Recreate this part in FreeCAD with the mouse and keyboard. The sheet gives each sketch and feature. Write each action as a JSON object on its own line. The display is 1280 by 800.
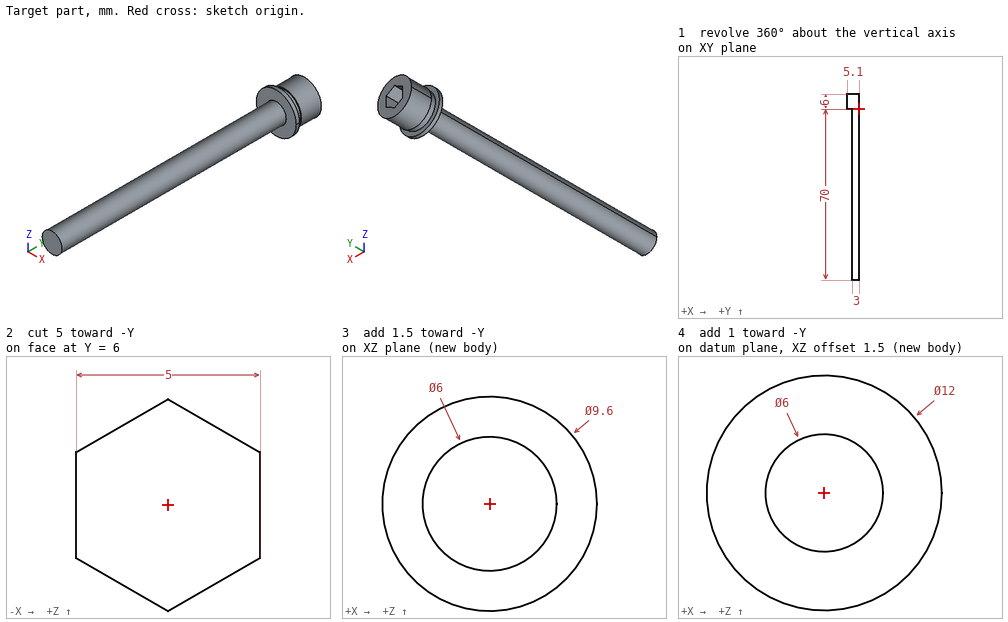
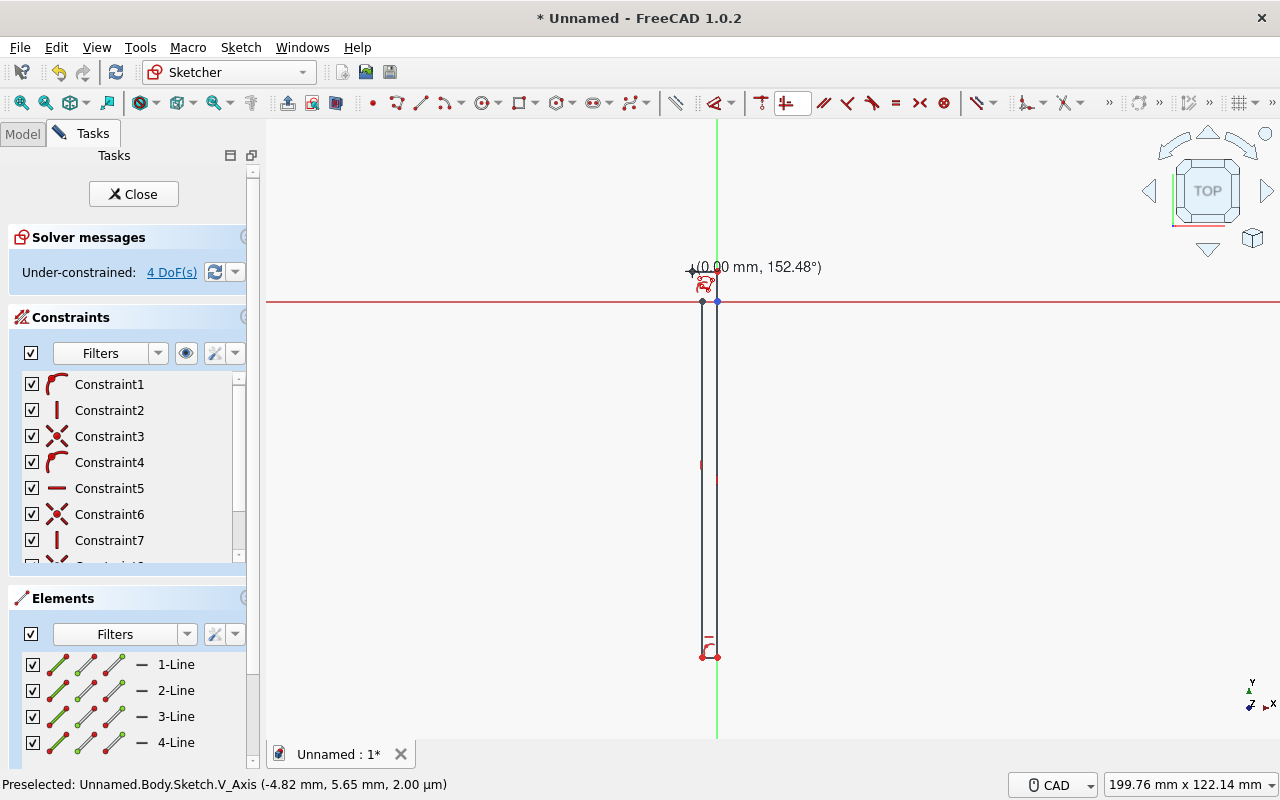
{"action": "scroll", "coordinate": [692, 302], "scroll_direction": "up", "scroll_amount": 2}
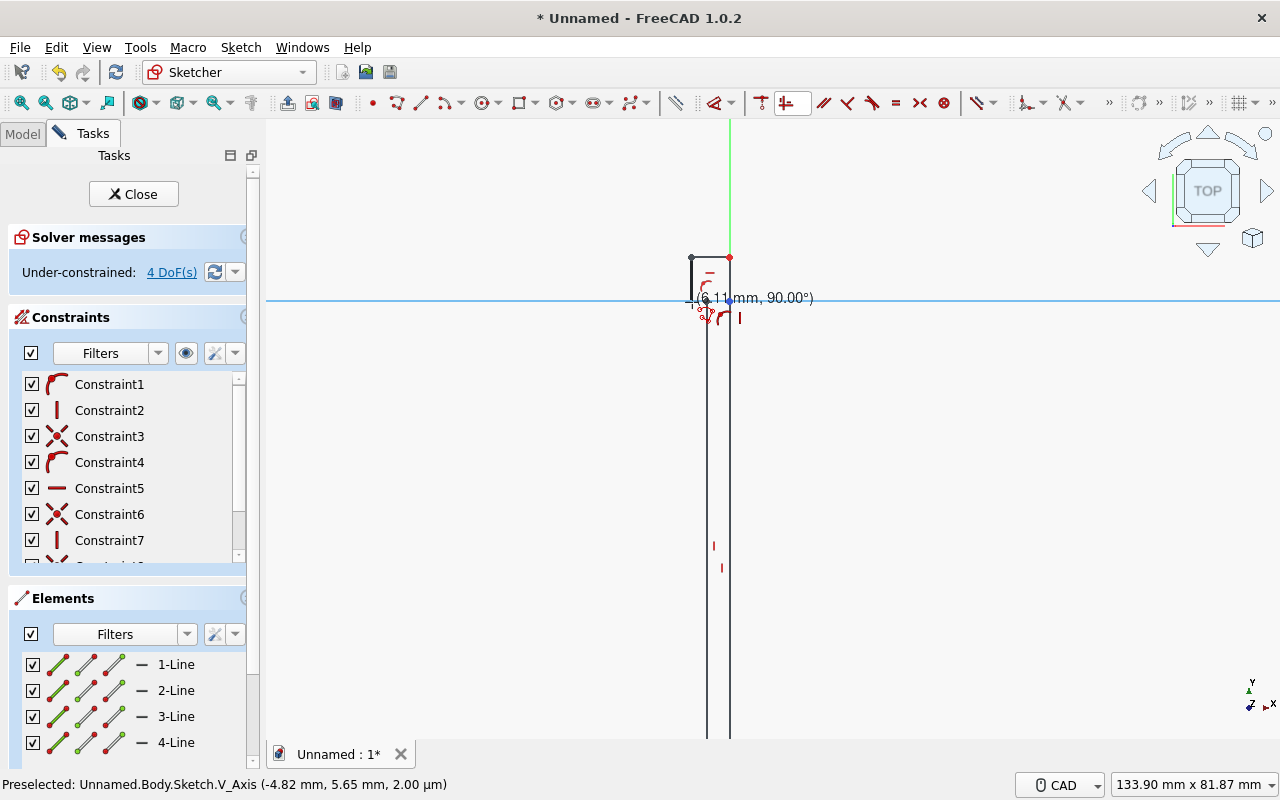
{"action": "left_click", "coordinate": [692, 310]}
{"action": "left_click", "coordinate": [707, 301]}
{"action": "key", "text": "Escape"}
{"action": "key", "text": "Escape"}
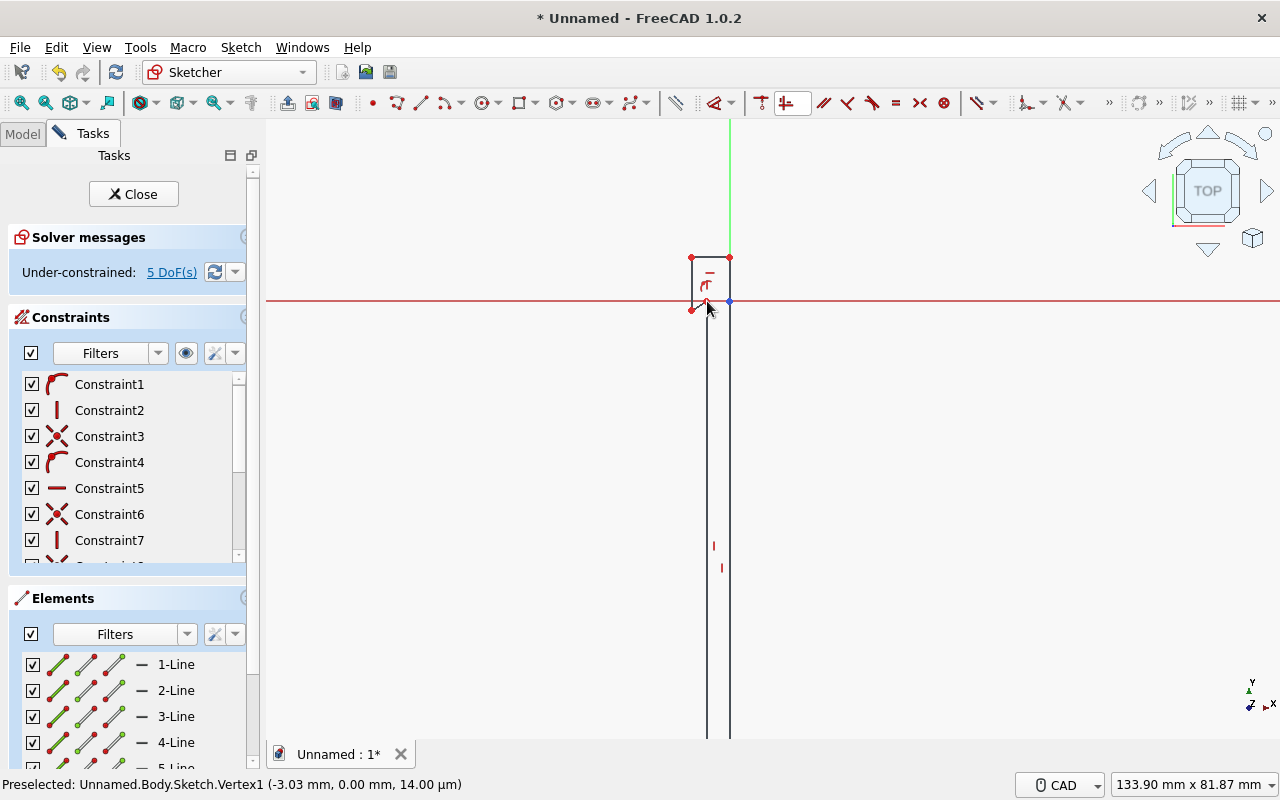
{"action": "scroll", "coordinate": [701, 305], "scroll_direction": "up", "scroll_amount": 5}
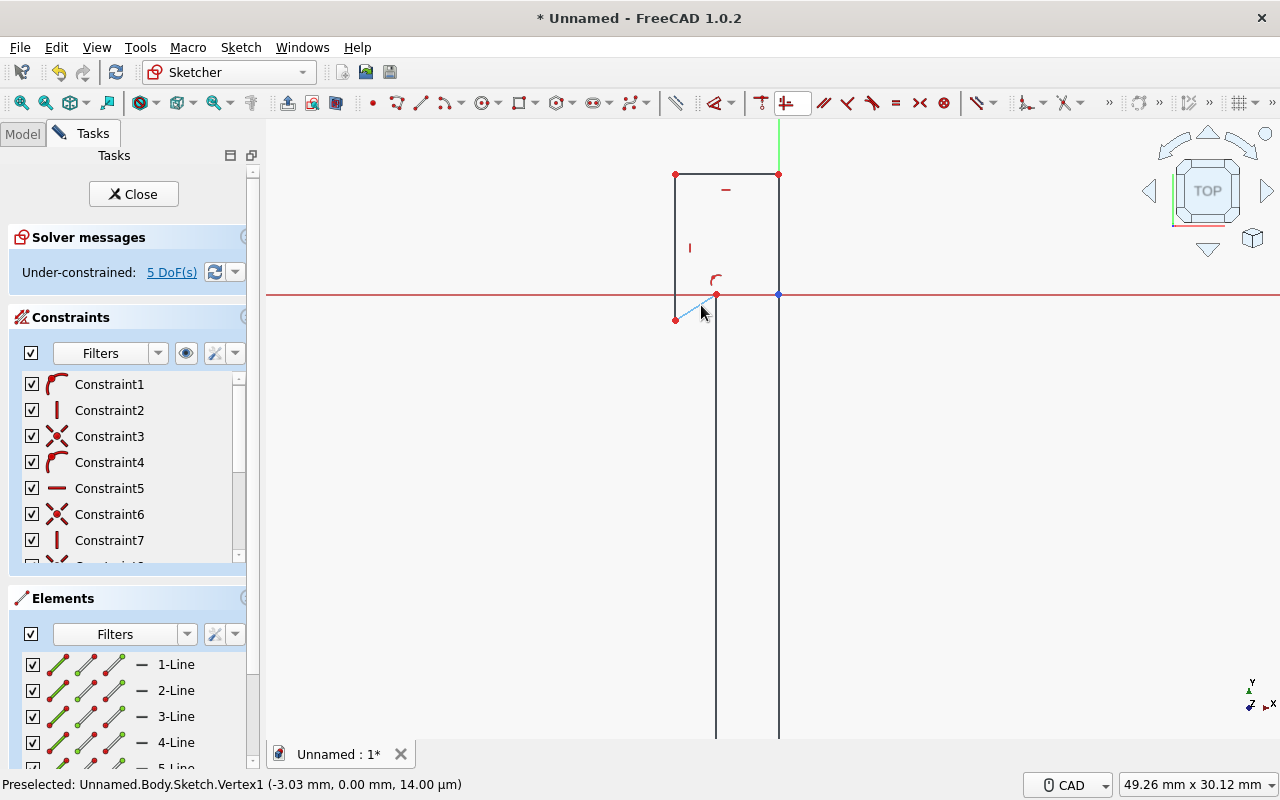
{"action": "left_click", "coordinate": [700, 305]}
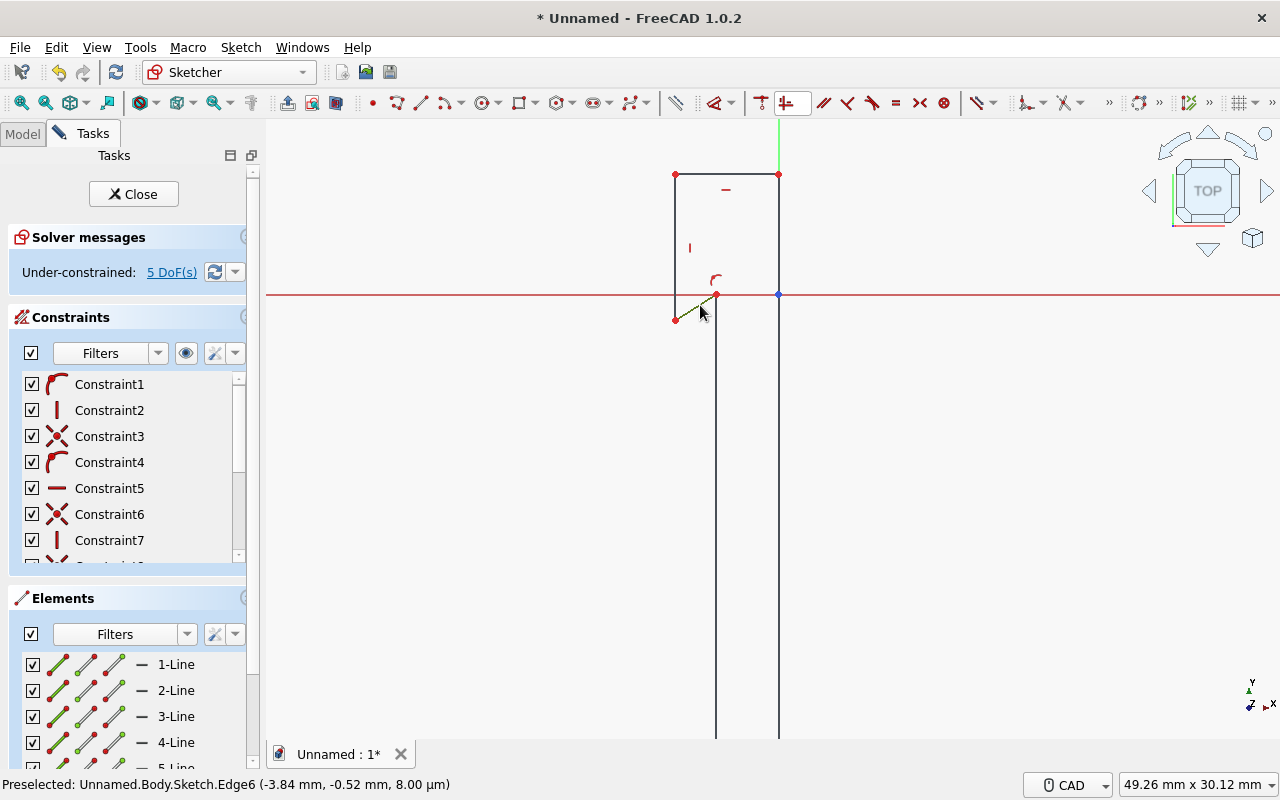
{"action": "key", "text": "h"}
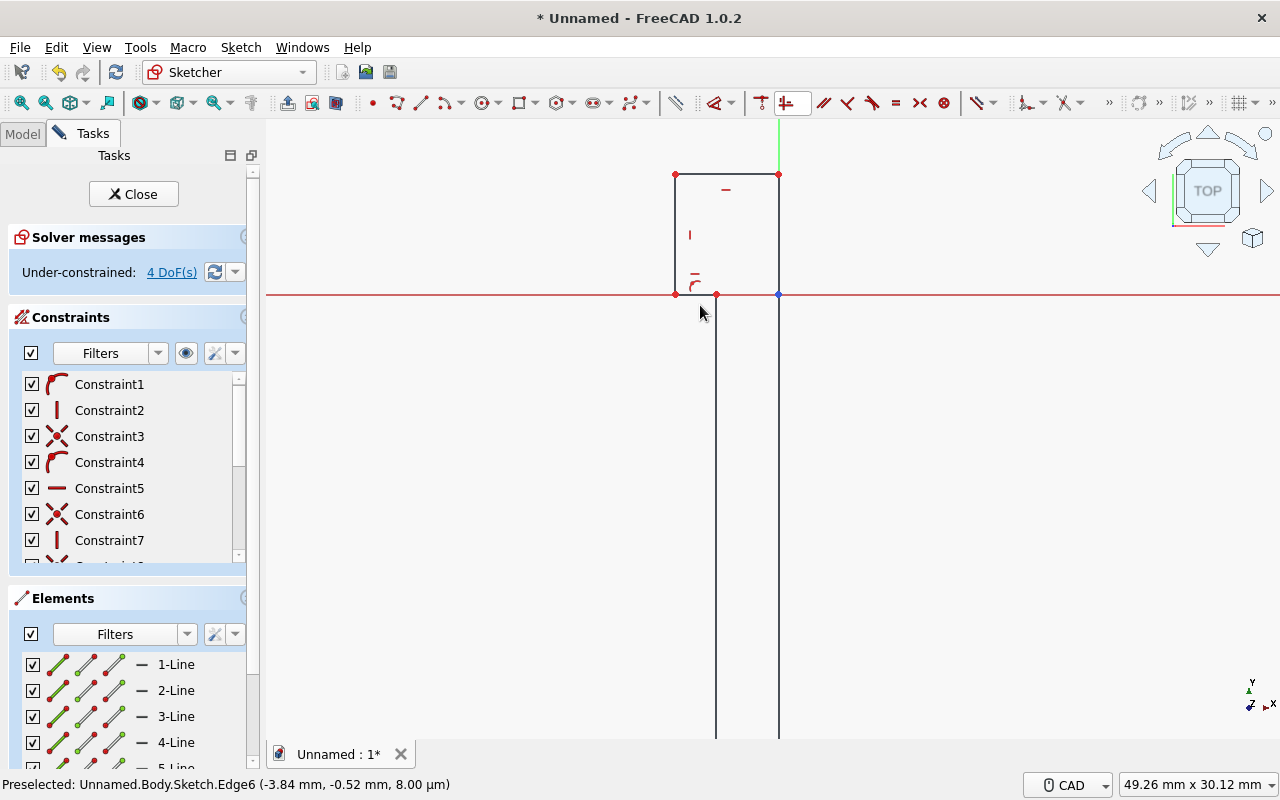
{"action": "scroll", "coordinate": [697, 257], "scroll_direction": "down", "scroll_amount": 7}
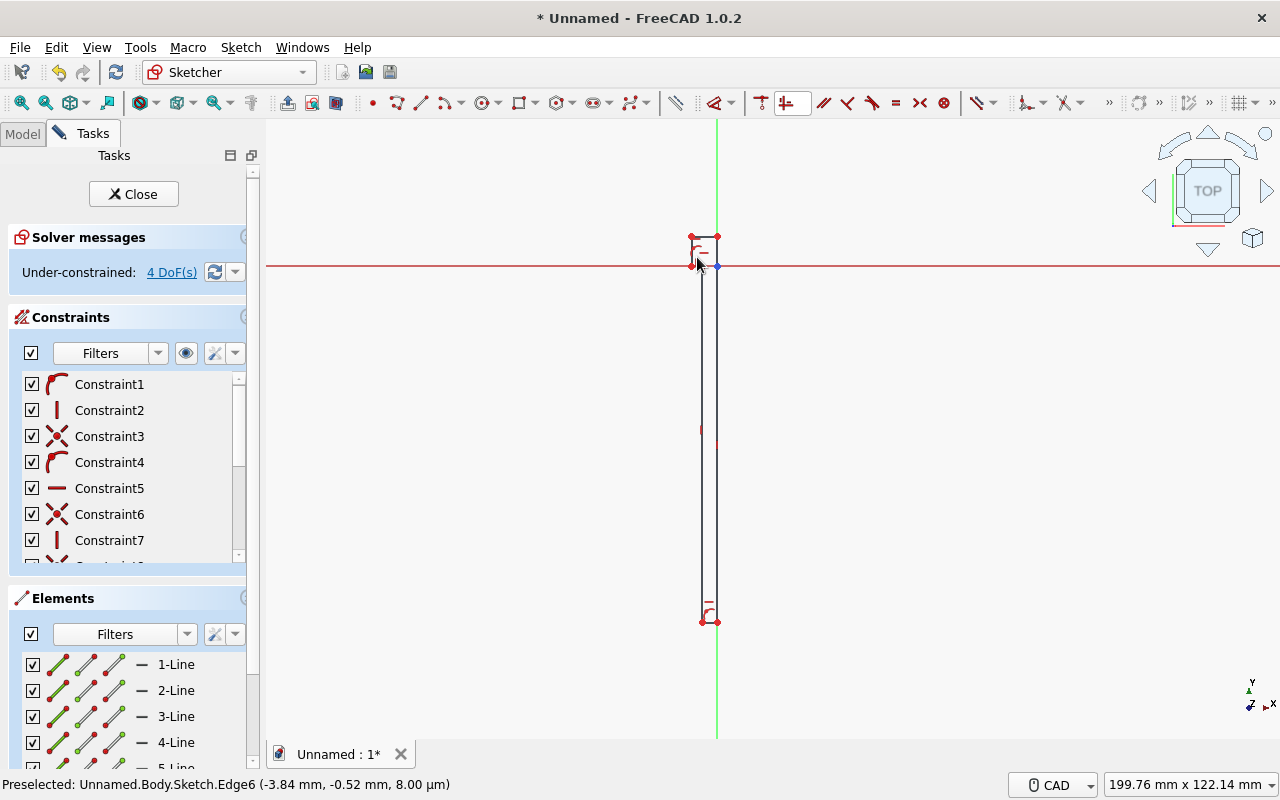
{"action": "scroll", "coordinate": [707, 623], "scroll_direction": "up", "scroll_amount": 6}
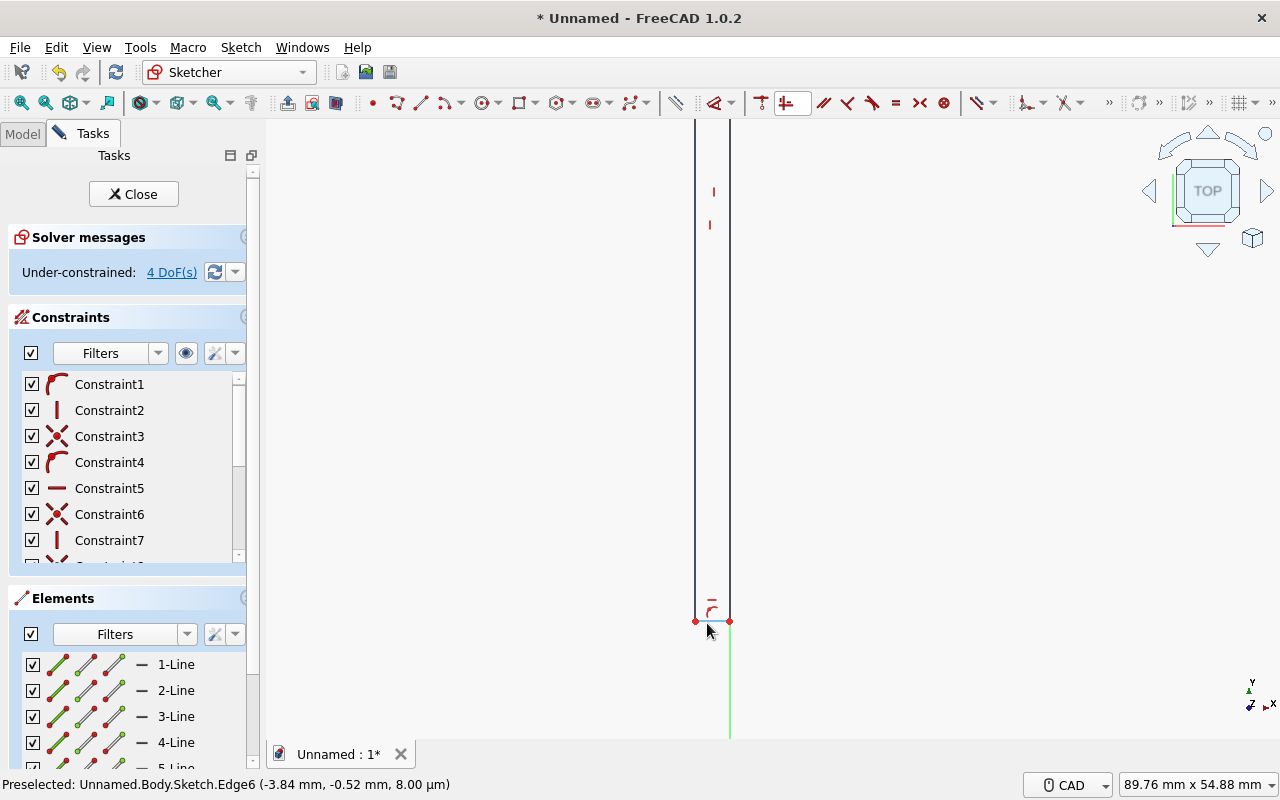
{"action": "left_click", "coordinate": [705, 620]}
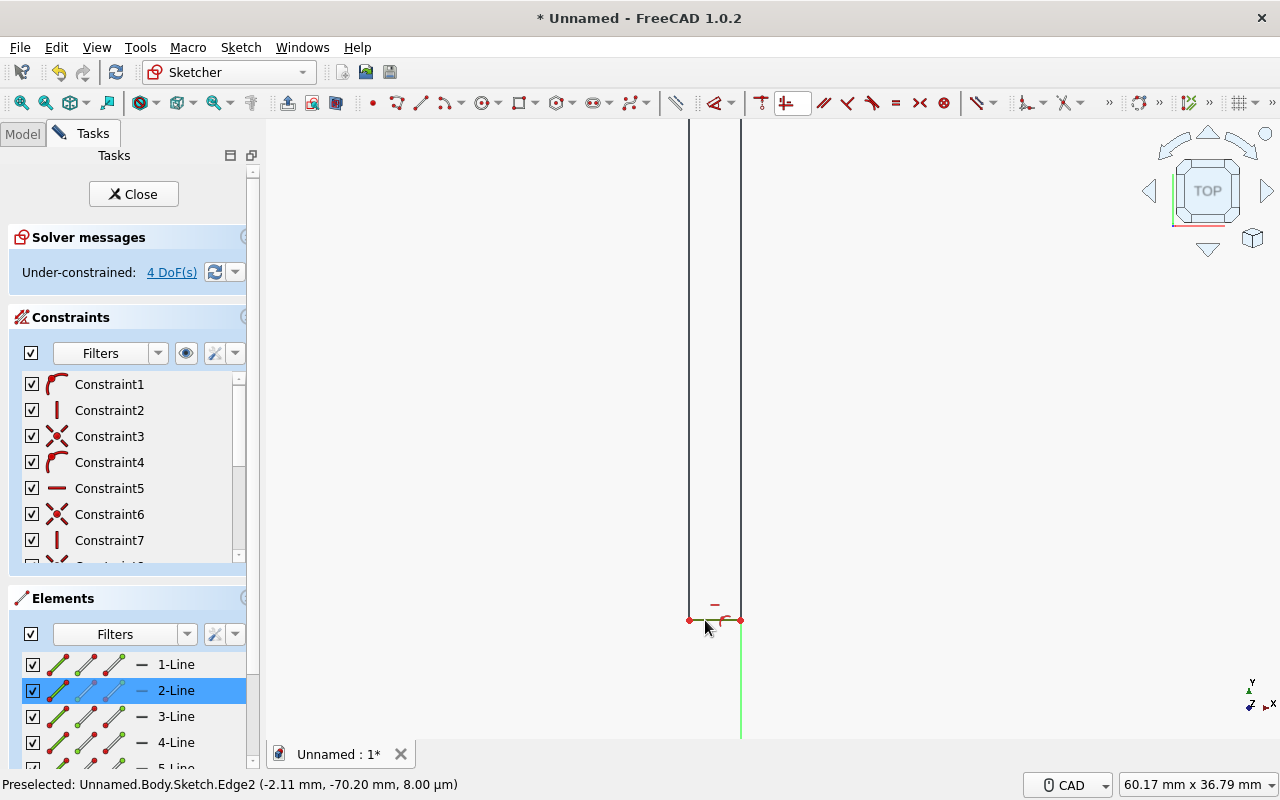
{"action": "left_click", "coordinate": [734, 104]}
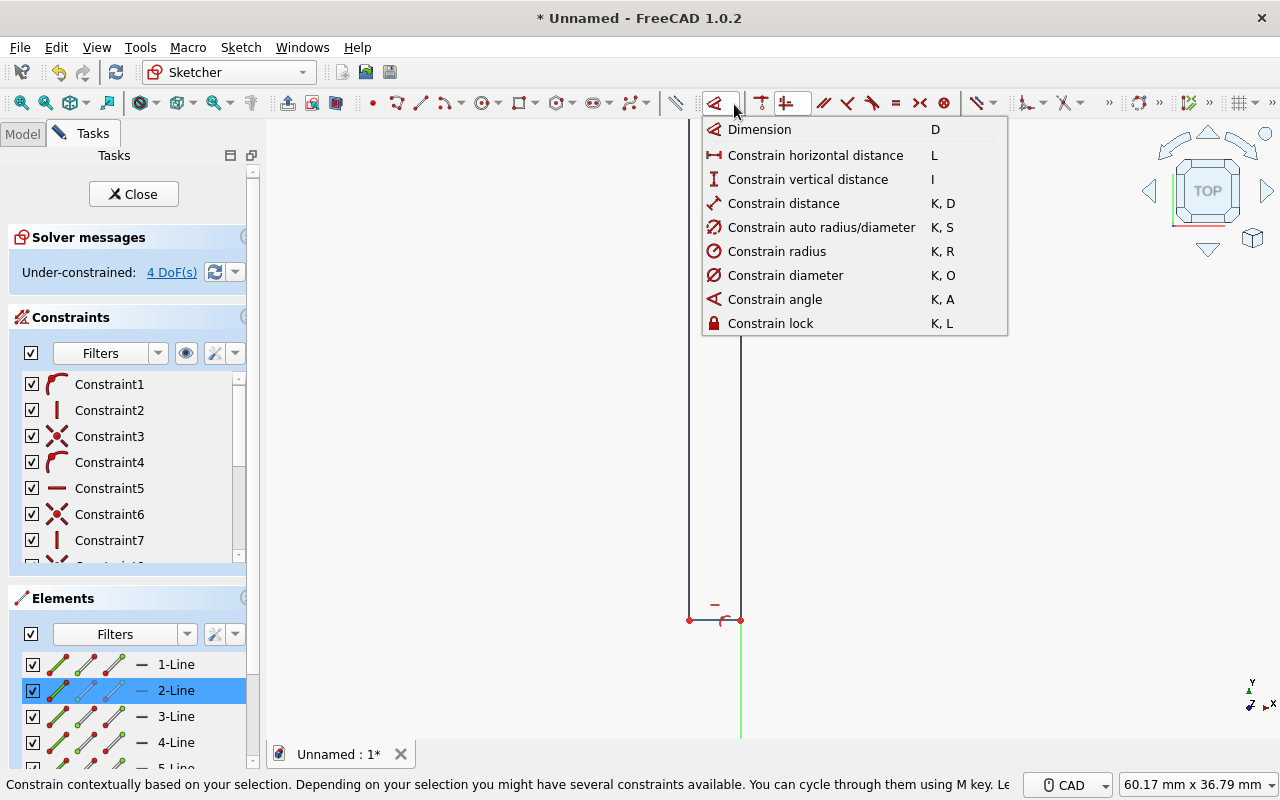
{"action": "left_click", "coordinate": [855, 155]}